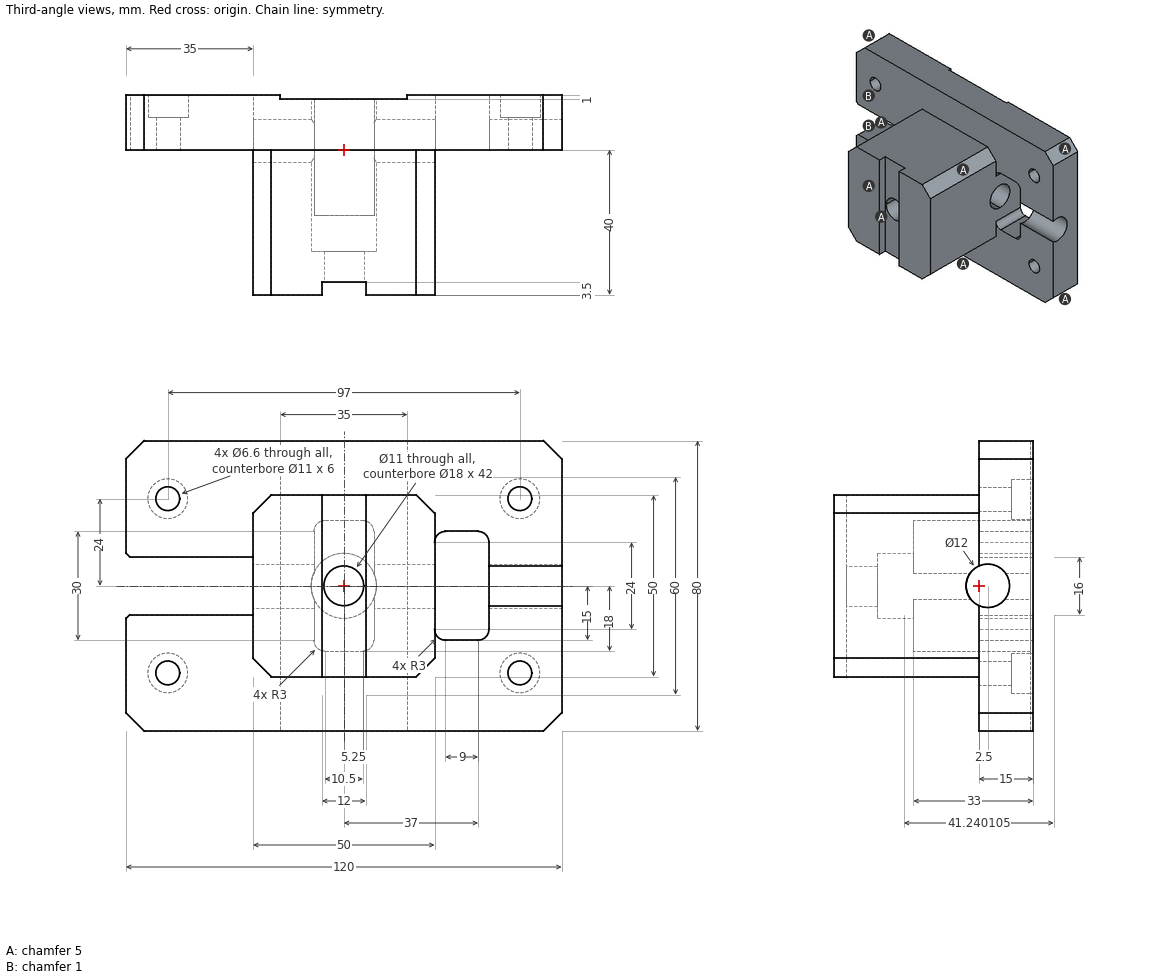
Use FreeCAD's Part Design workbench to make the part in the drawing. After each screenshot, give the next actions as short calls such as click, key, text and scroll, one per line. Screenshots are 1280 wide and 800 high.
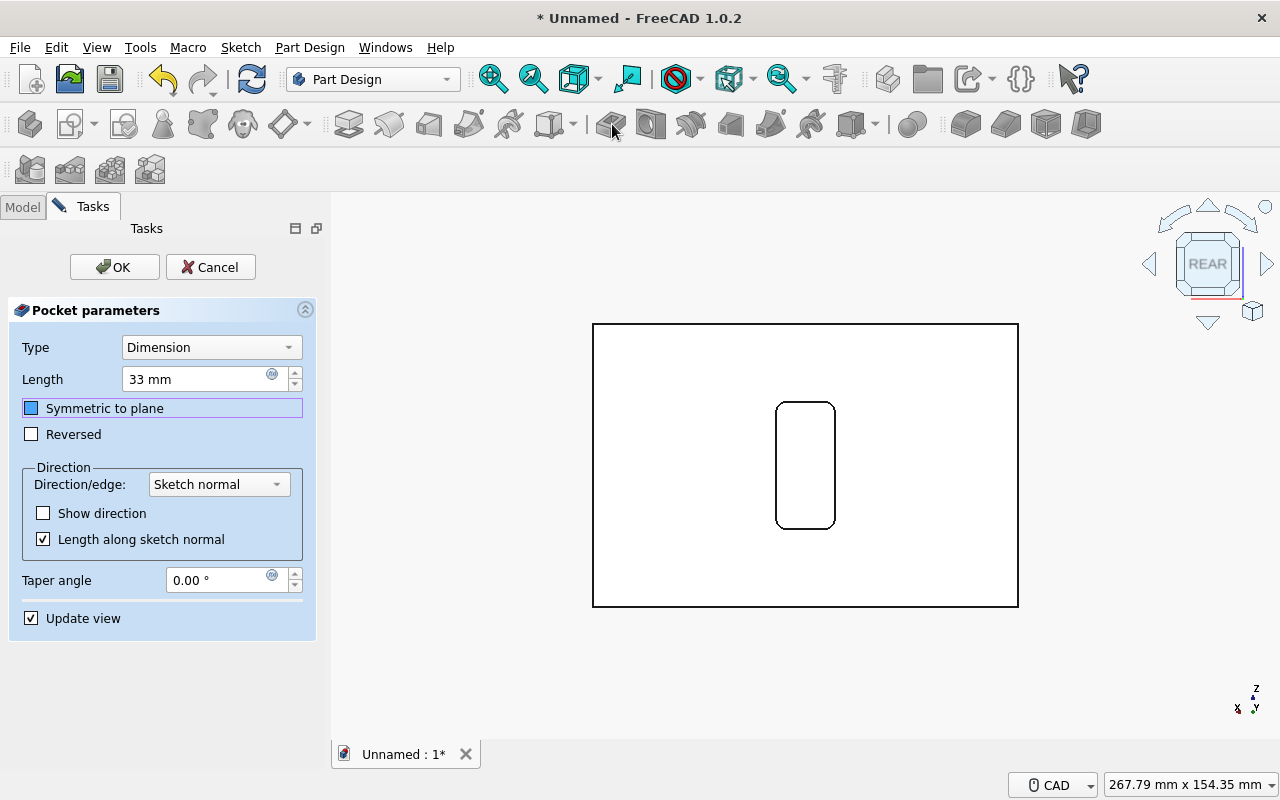
click(115, 267)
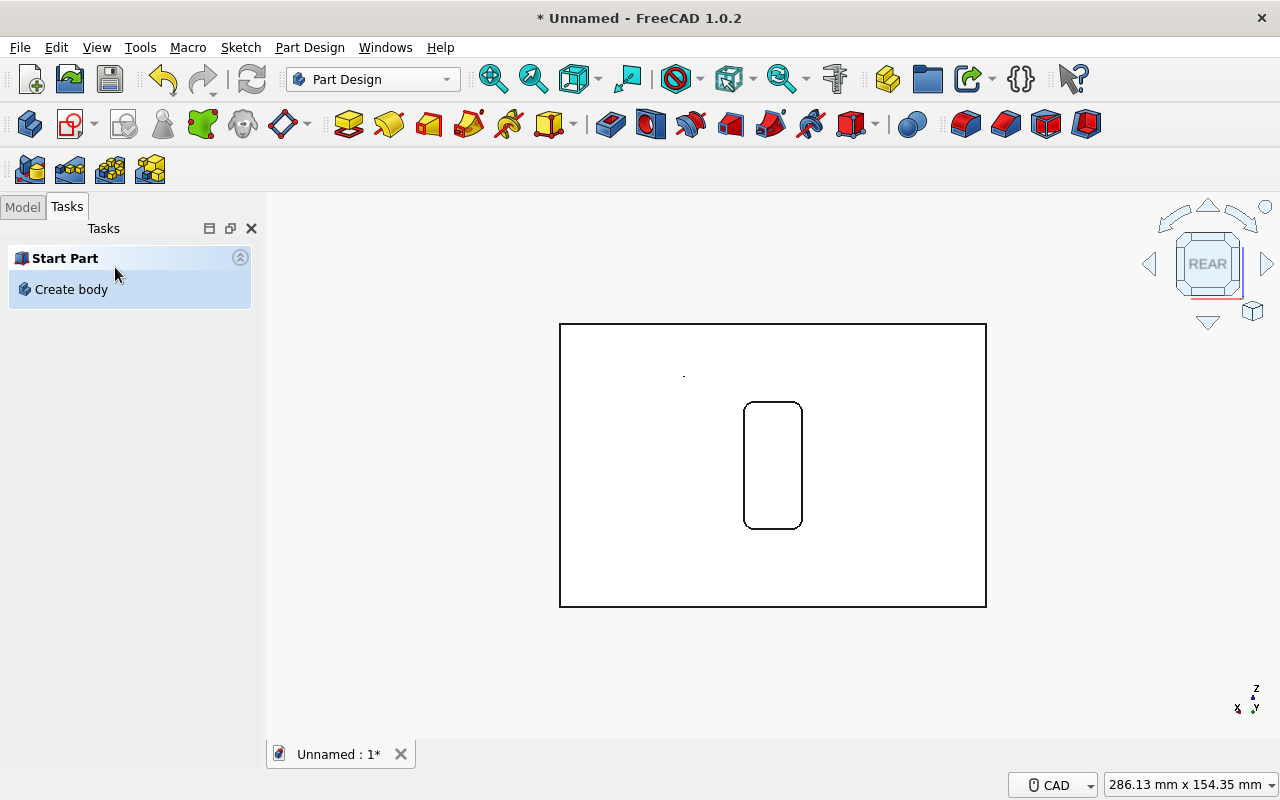
key(6)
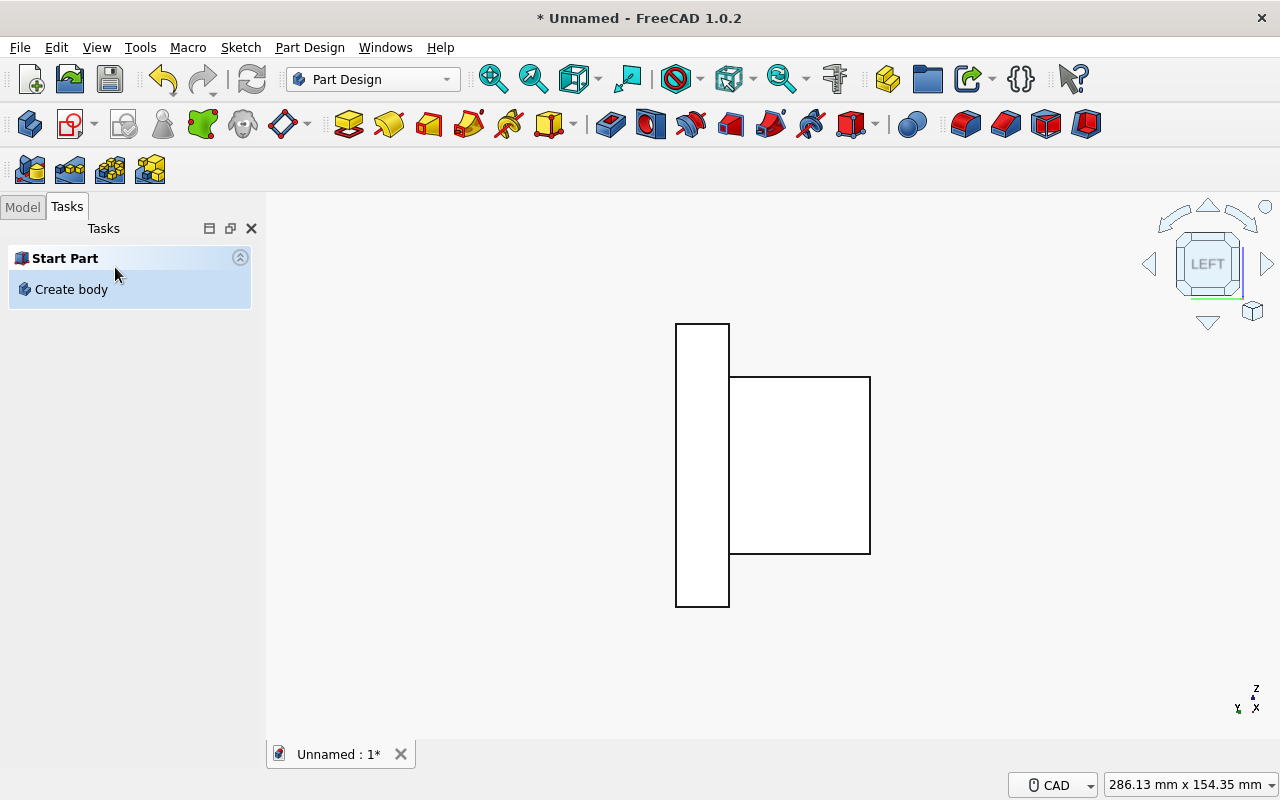
click(702, 465)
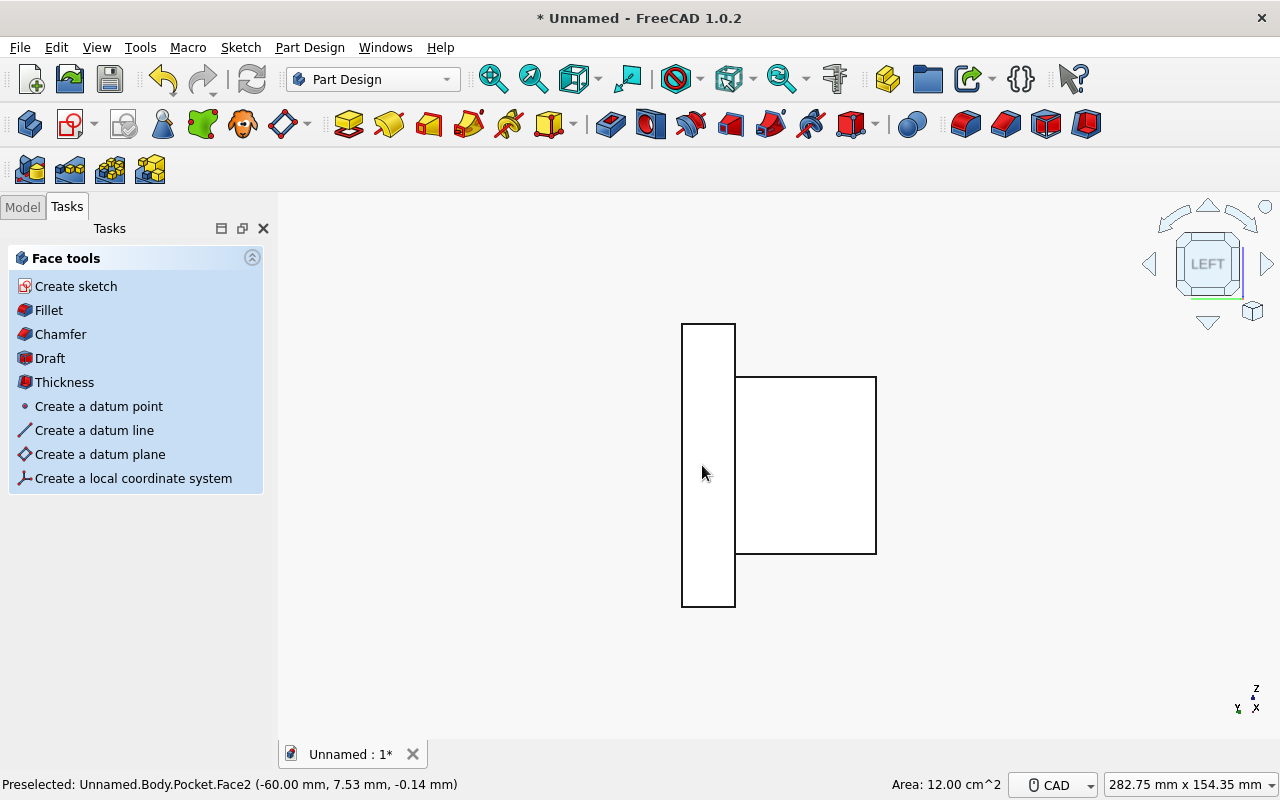
click(70, 124)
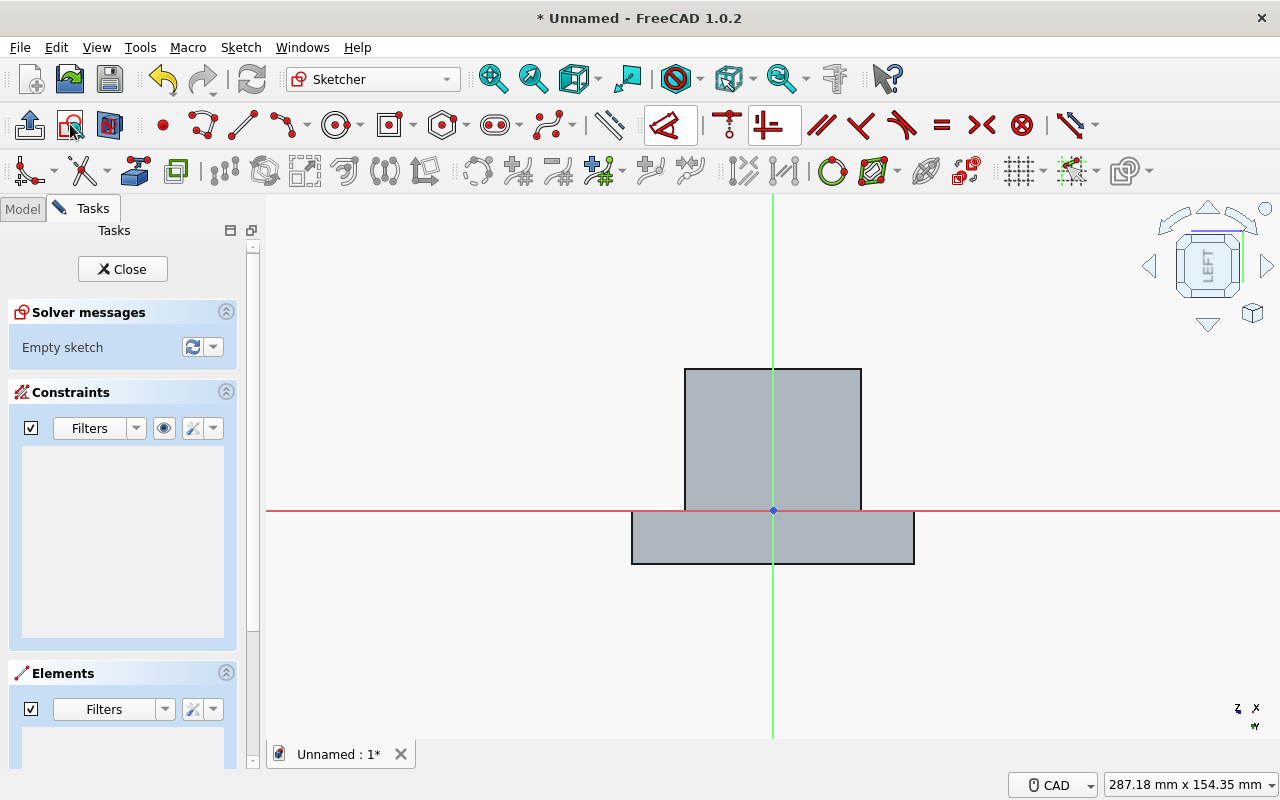
scroll(829, 547, up, 4)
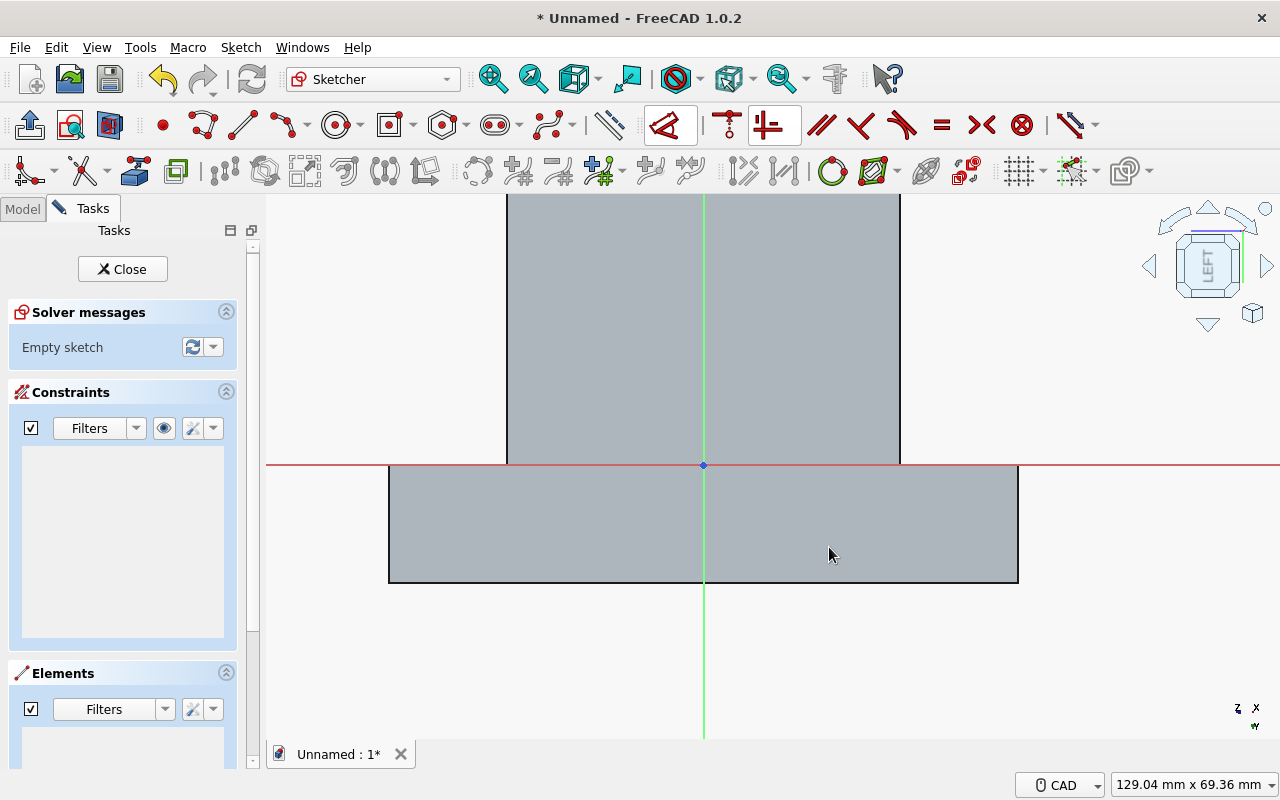
click(390, 126)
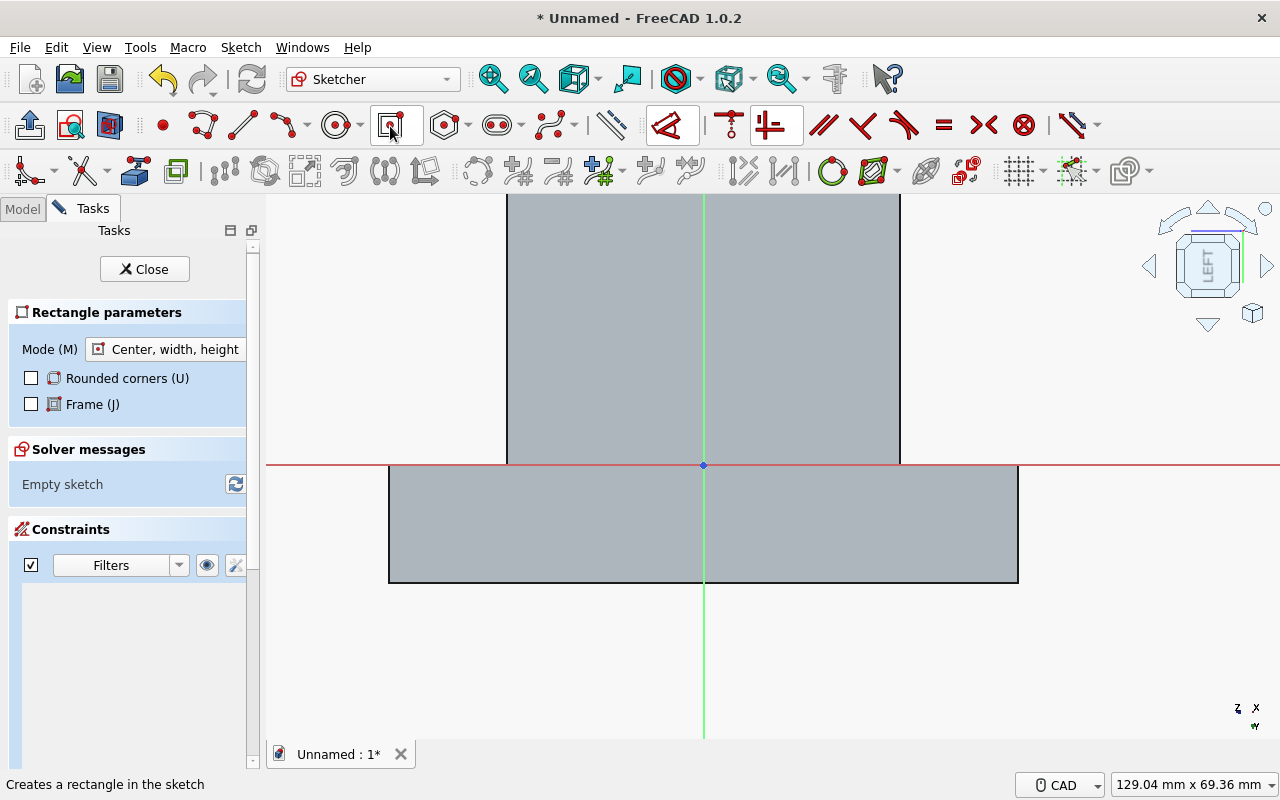
click(704, 465)
click(767, 303)
key(Escape)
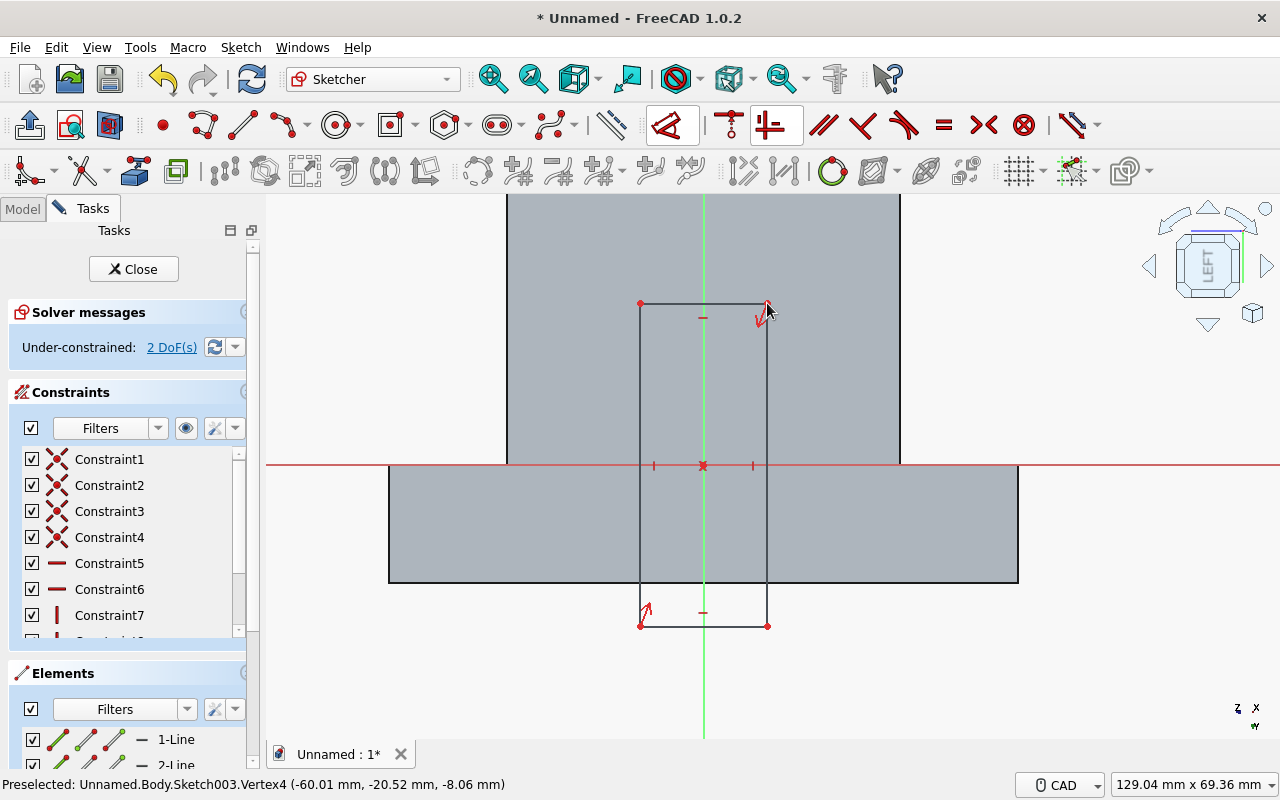
click(678, 627)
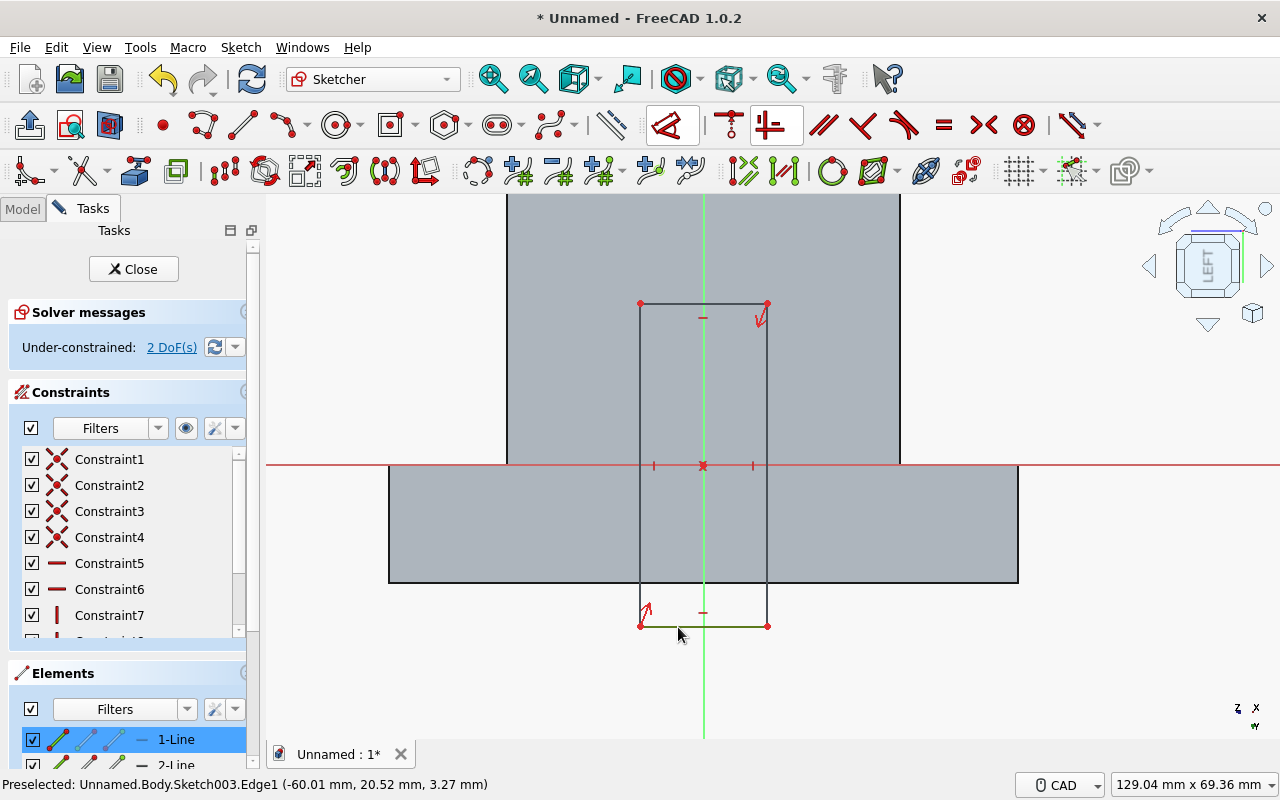
key(l)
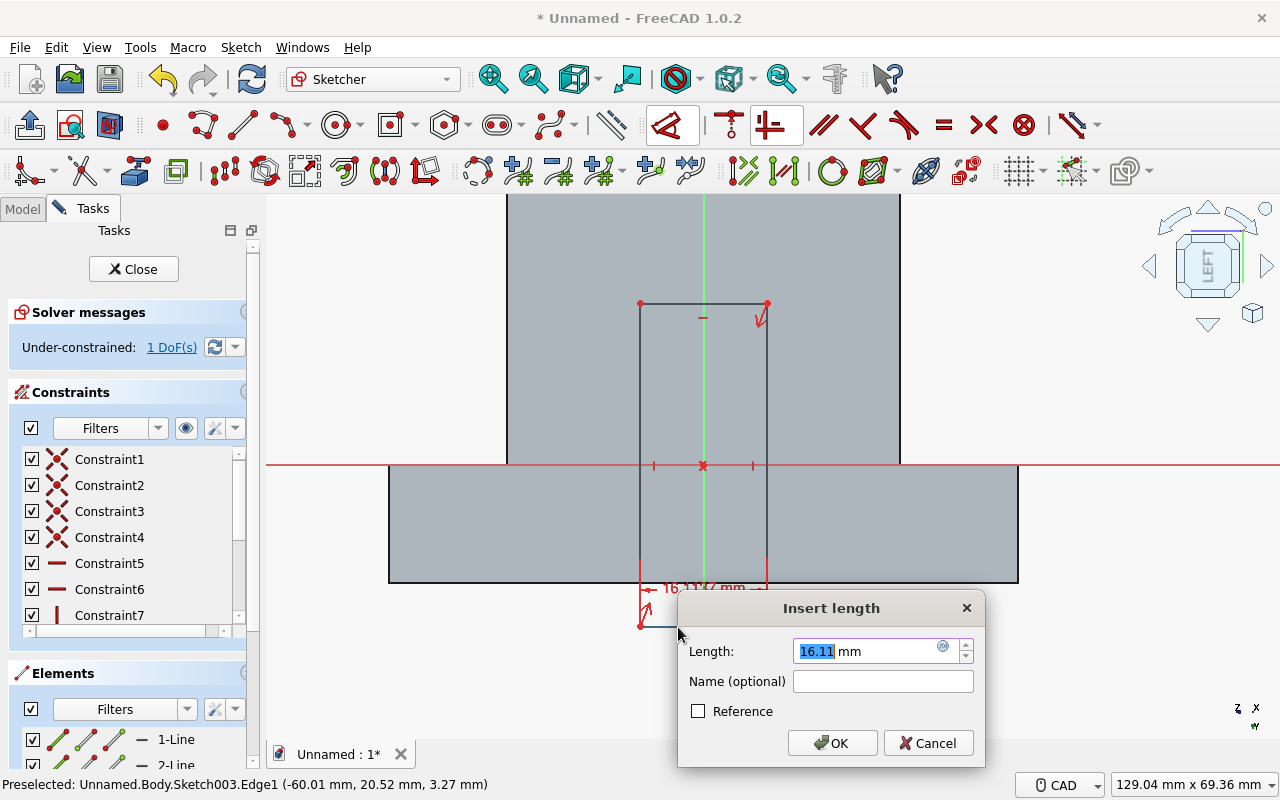
text(16)
key(Return)